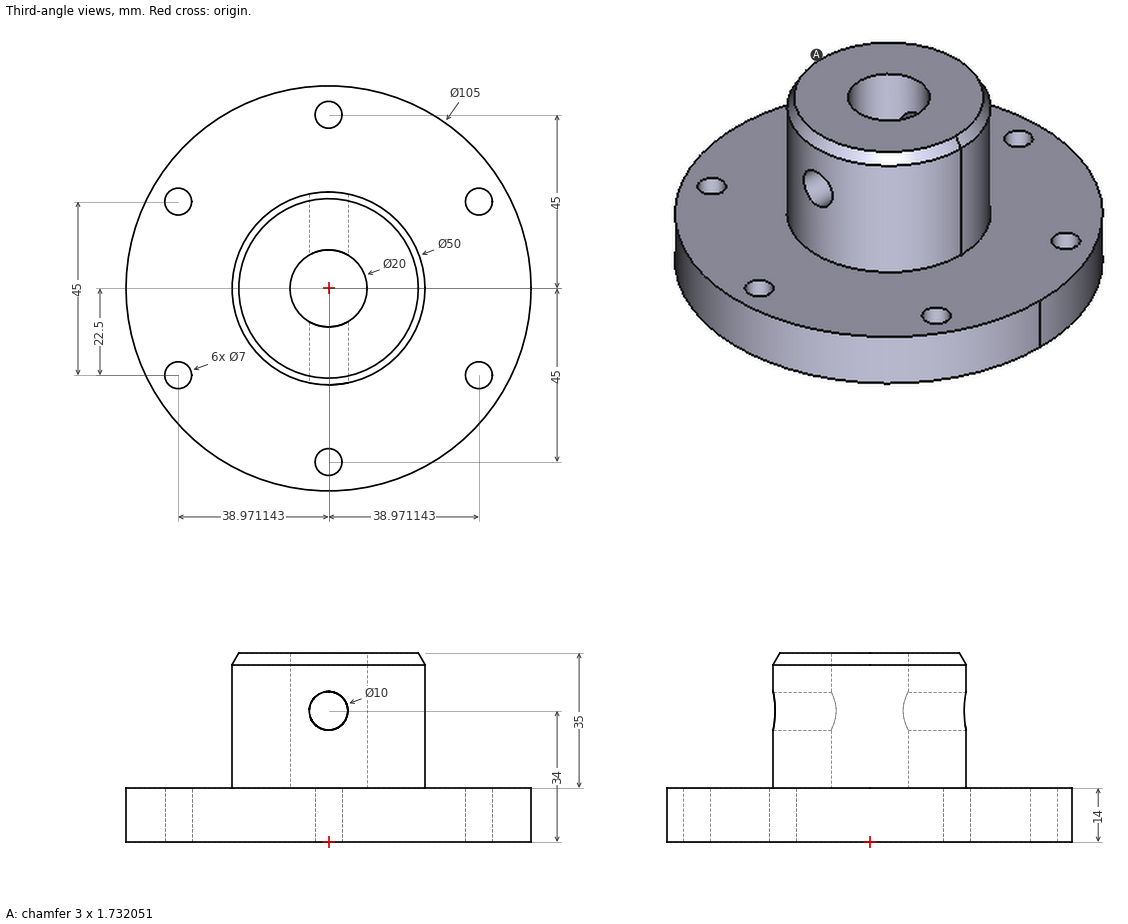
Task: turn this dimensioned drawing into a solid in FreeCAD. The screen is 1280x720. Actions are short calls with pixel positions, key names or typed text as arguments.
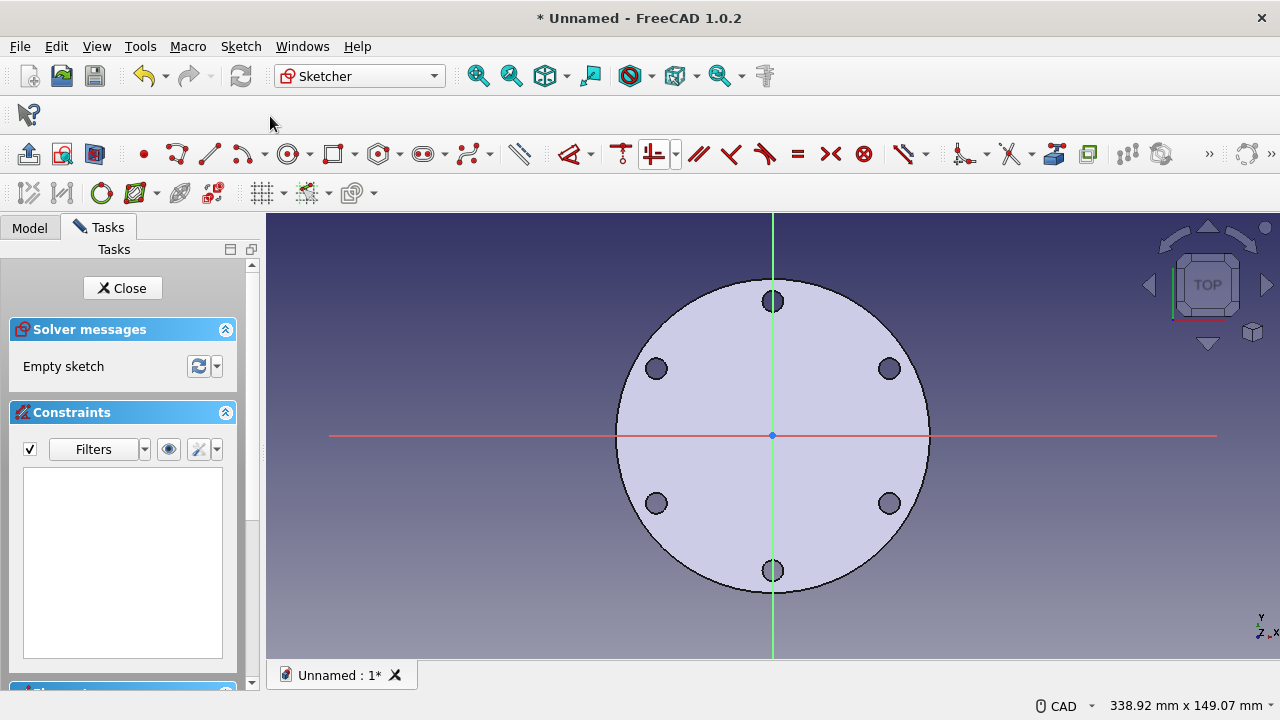
scroll(856, 436, up, 3)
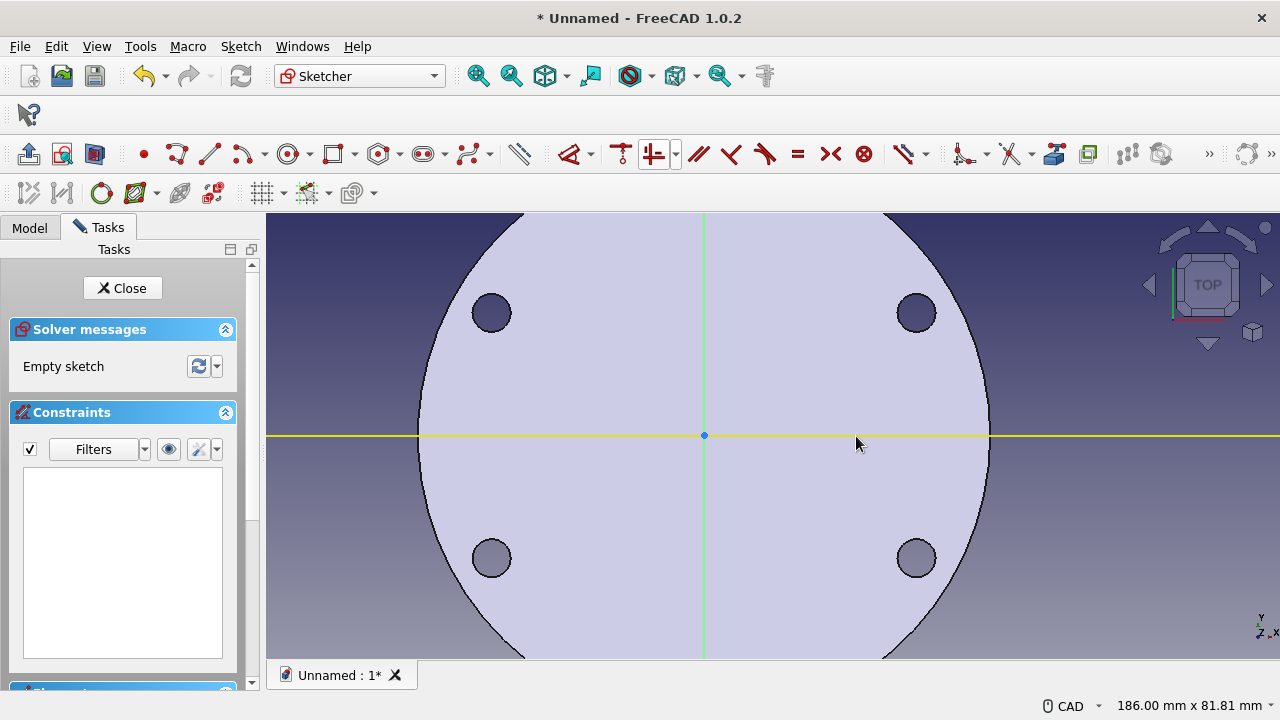
click(288, 154)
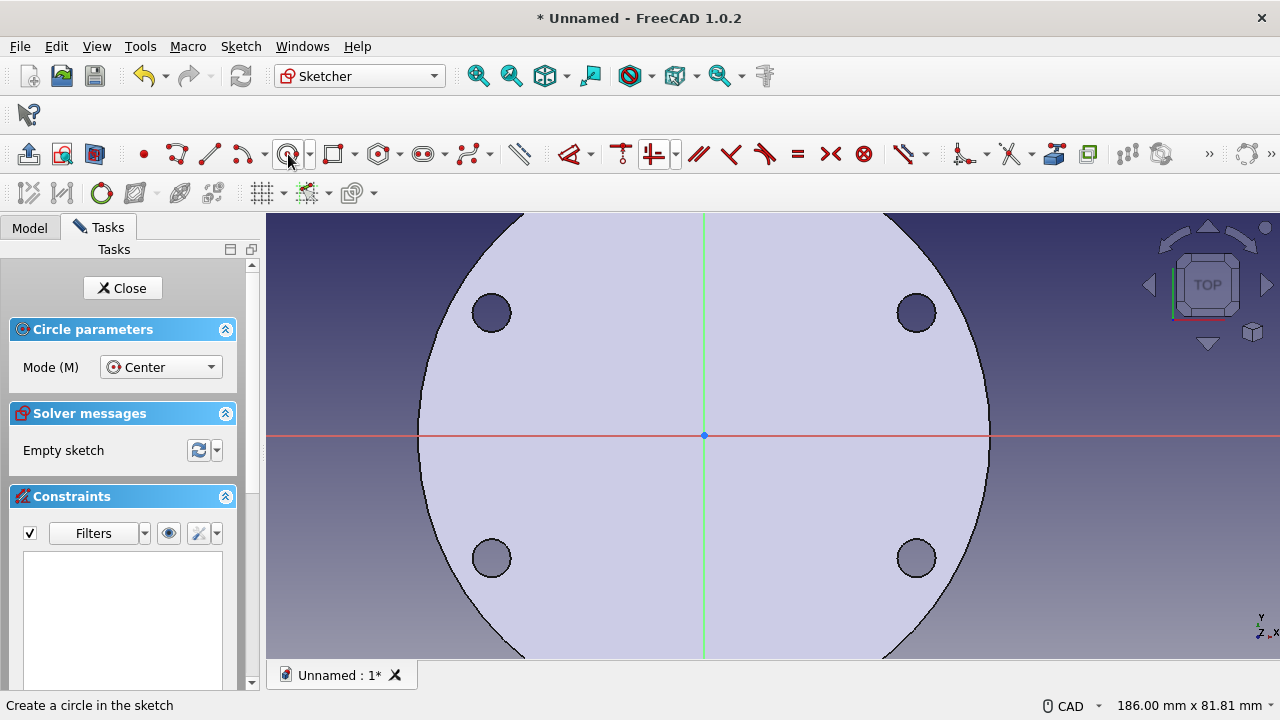
click(704, 436)
click(800, 339)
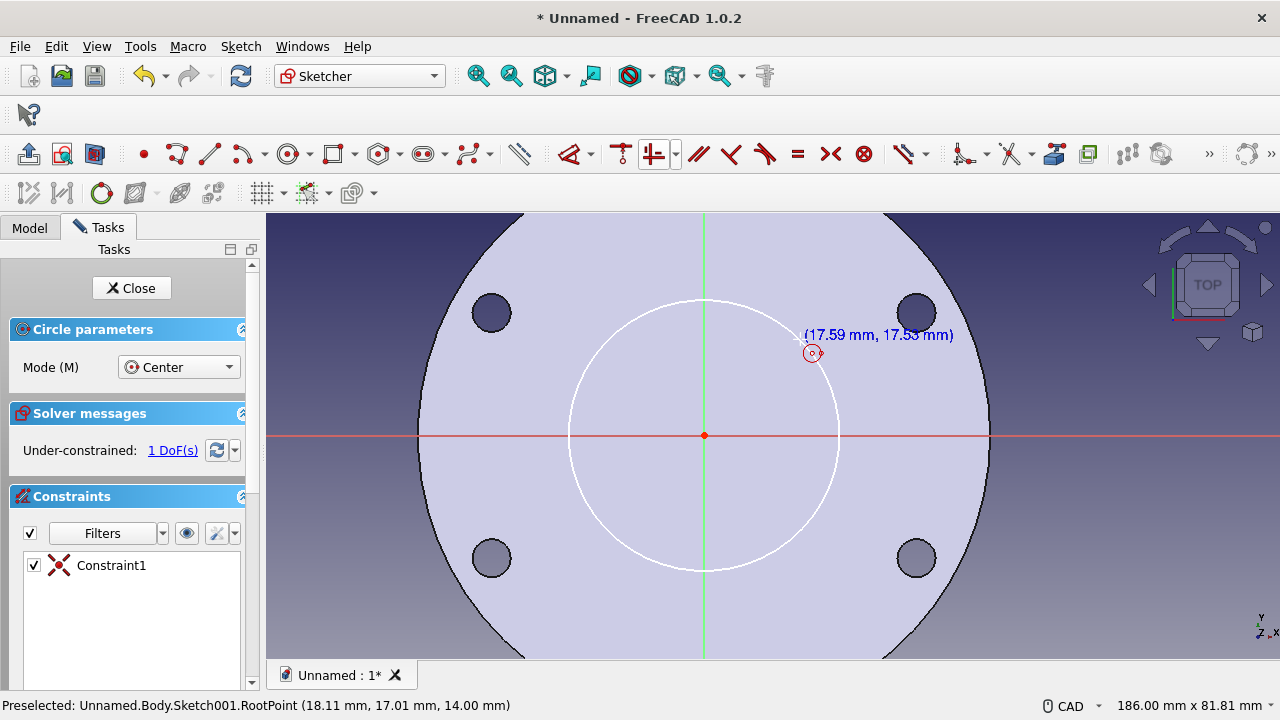
click(704, 436)
click(743, 397)
key(Escape)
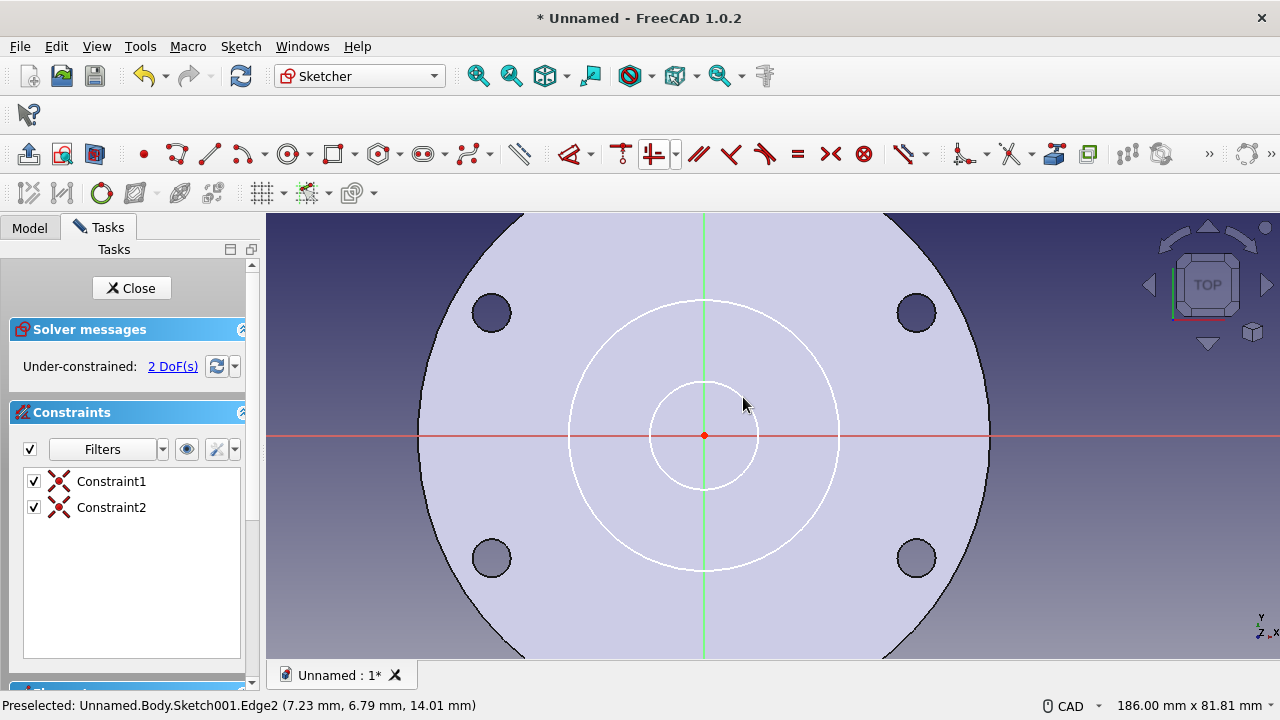
click(568, 154)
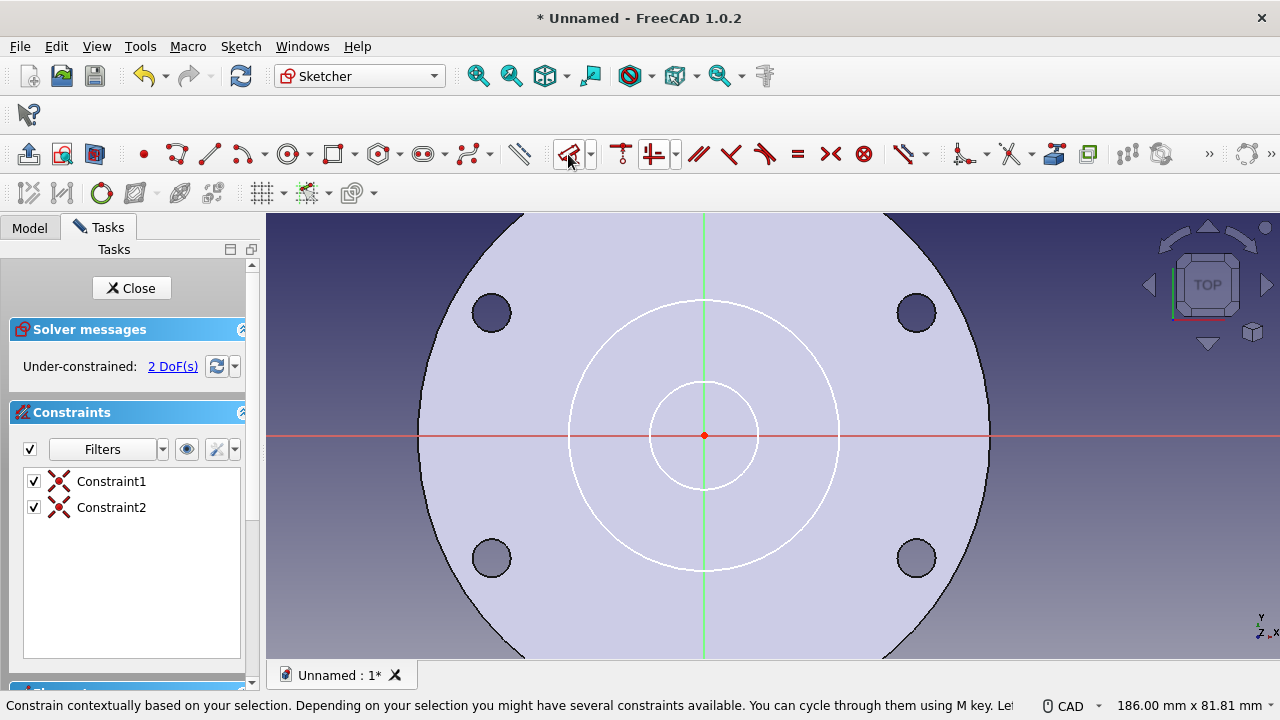
click(800, 340)
click(823, 317)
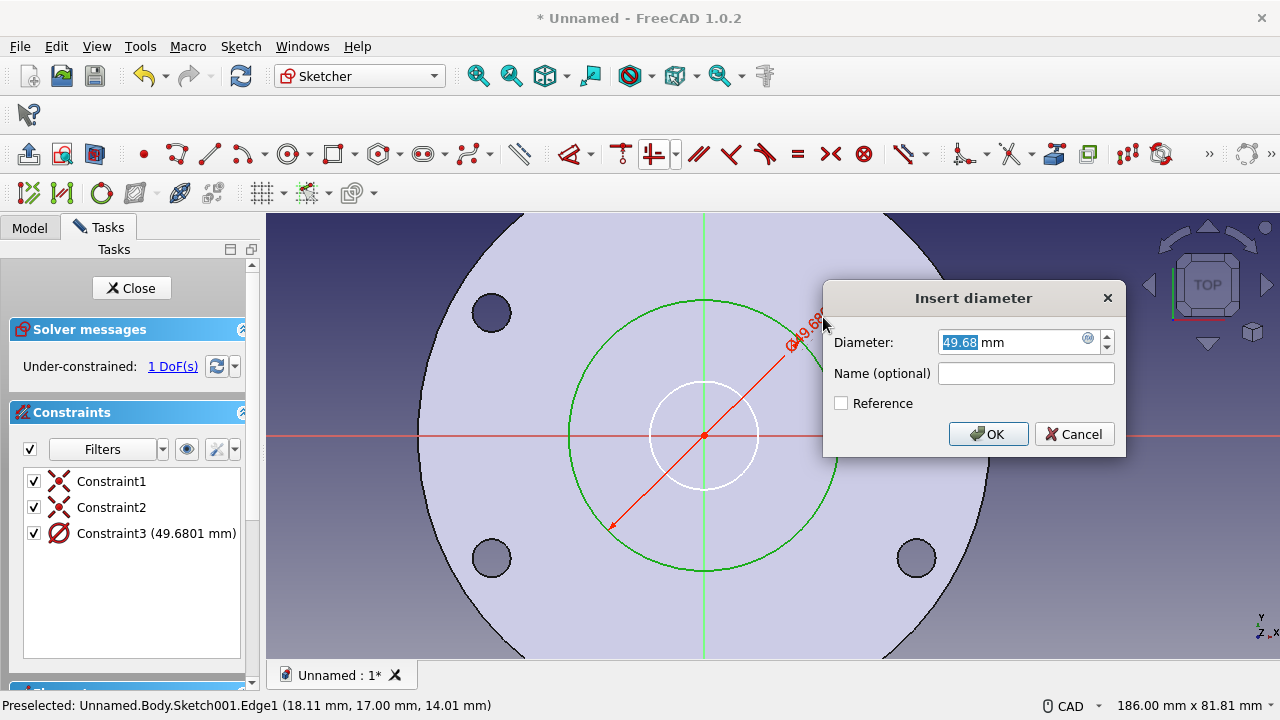
text(50)
key(Return)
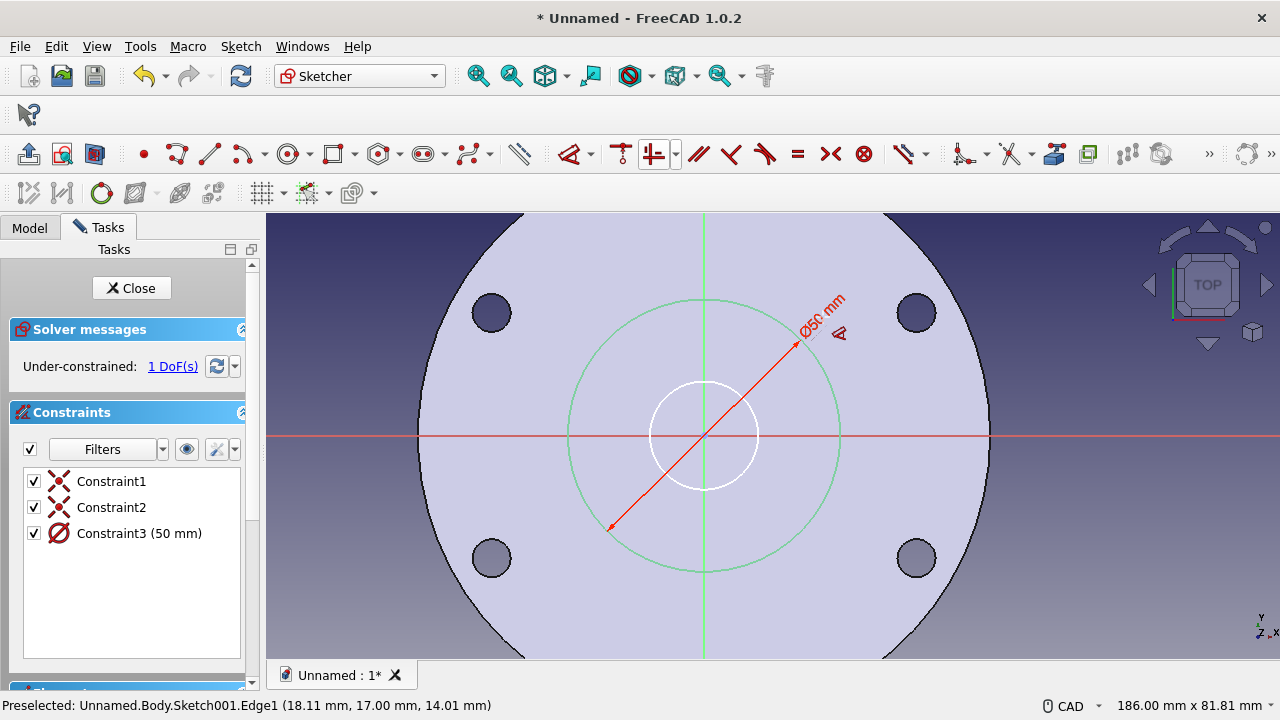
click(742, 397)
click(764, 374)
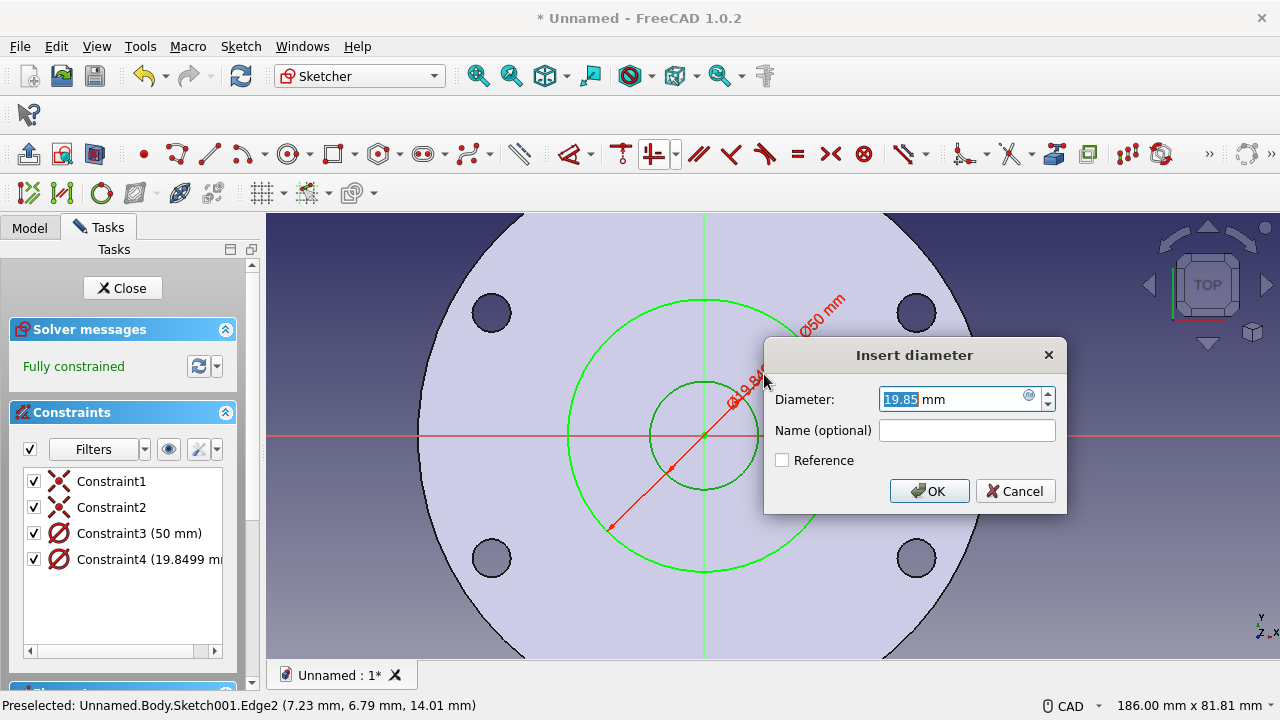
text(20)
key(Return)
key(Escape)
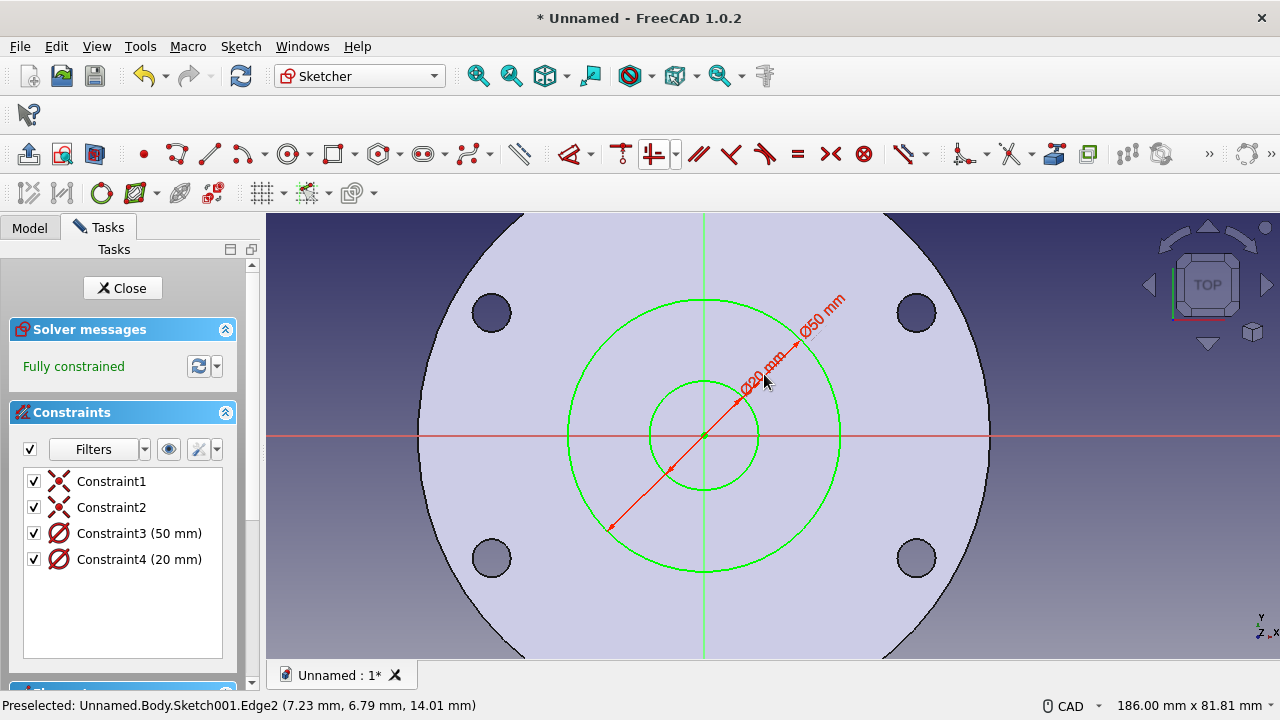
click(123, 288)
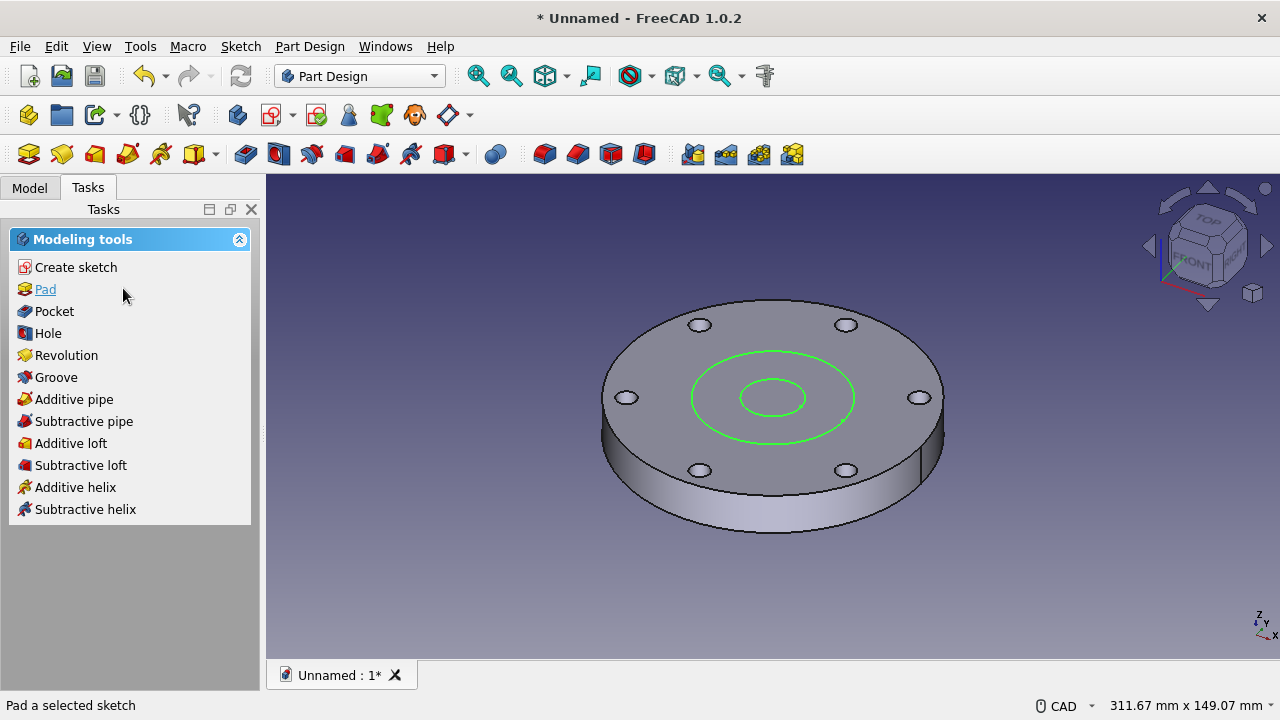
click(29, 154)